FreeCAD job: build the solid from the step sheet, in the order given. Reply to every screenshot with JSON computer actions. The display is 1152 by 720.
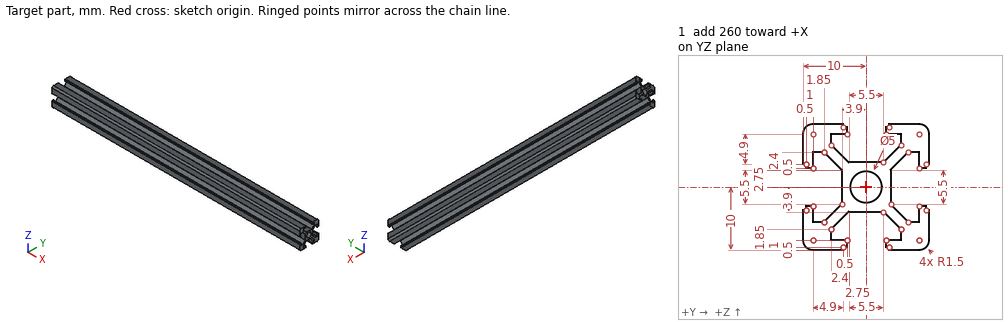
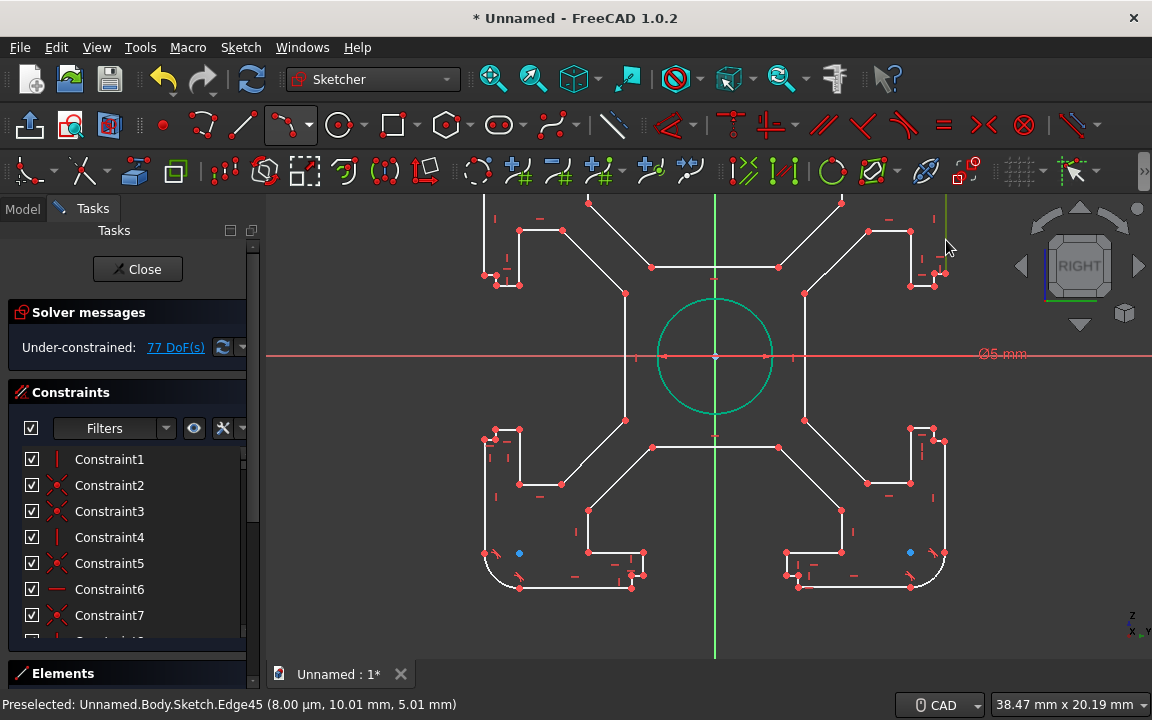
{"action": "scroll", "coordinate": [489, 569], "scroll_direction": "down", "scroll_amount": 2}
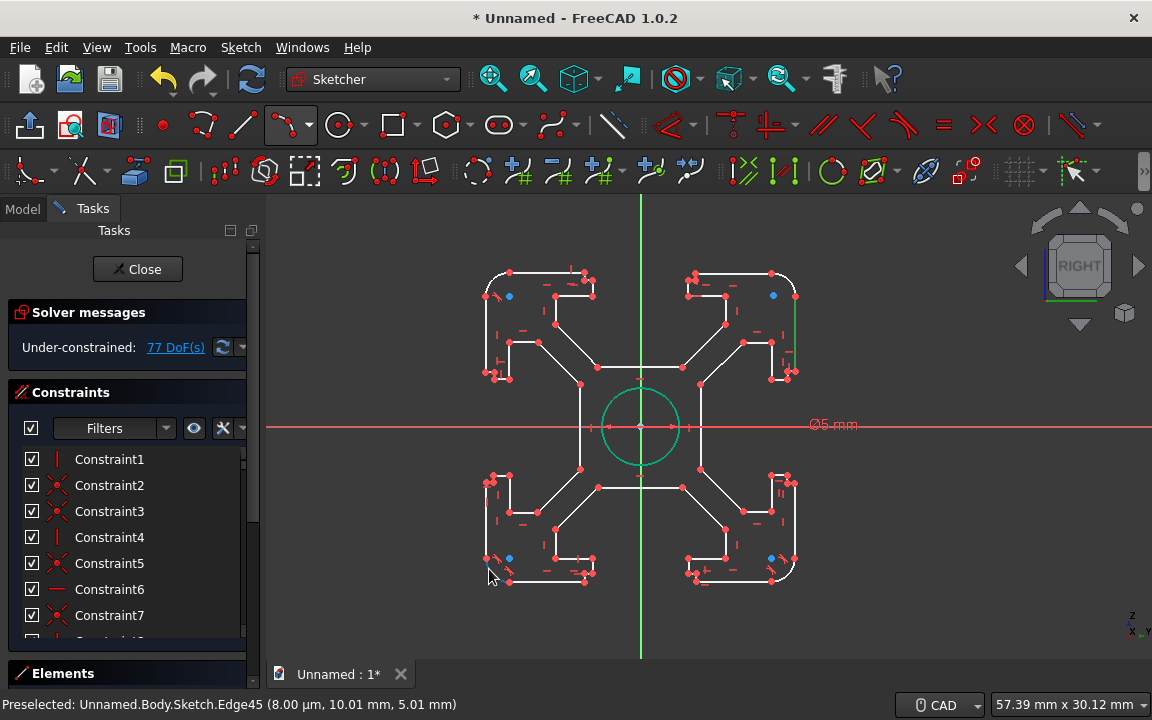
{"action": "scroll", "coordinate": [793, 286], "scroll_direction": "up", "scroll_amount": 2}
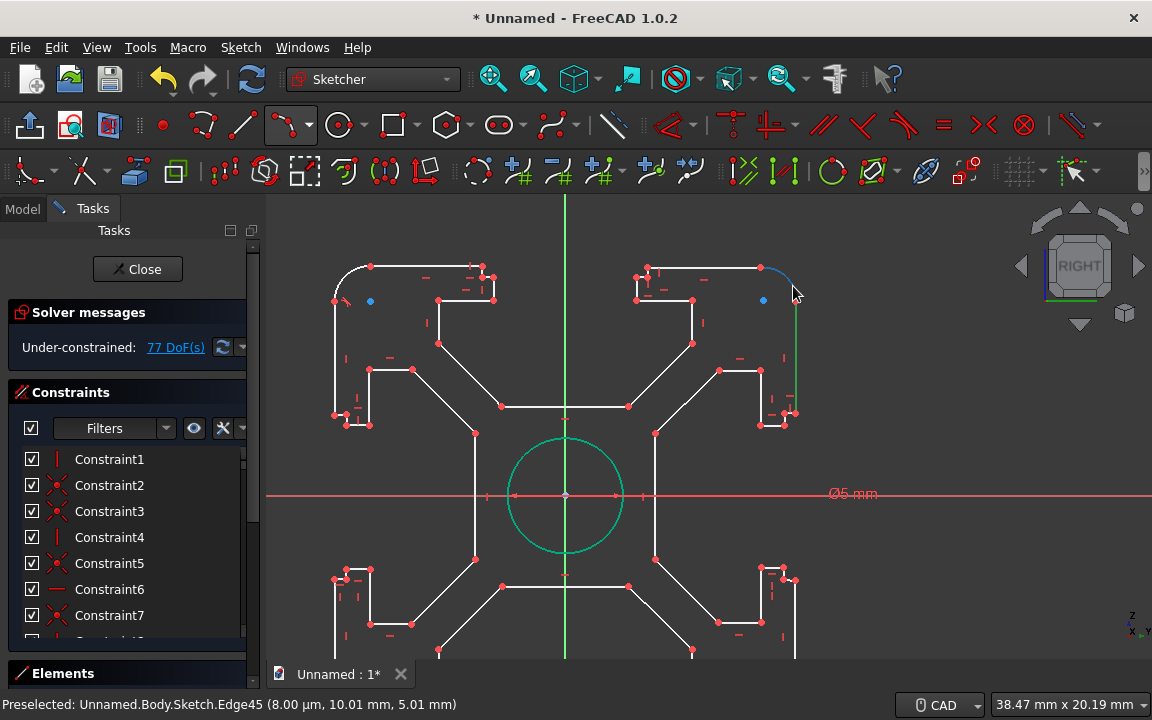
{"action": "left_click", "coordinate": [793, 286]}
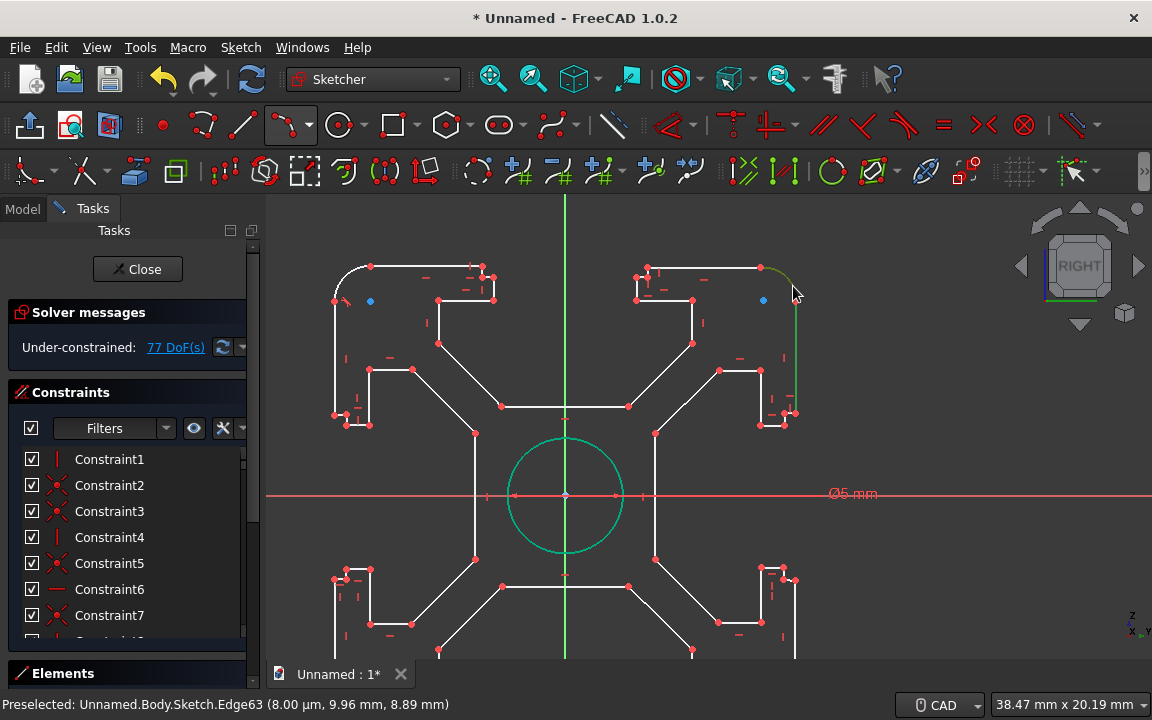
{"action": "key", "text": "t"}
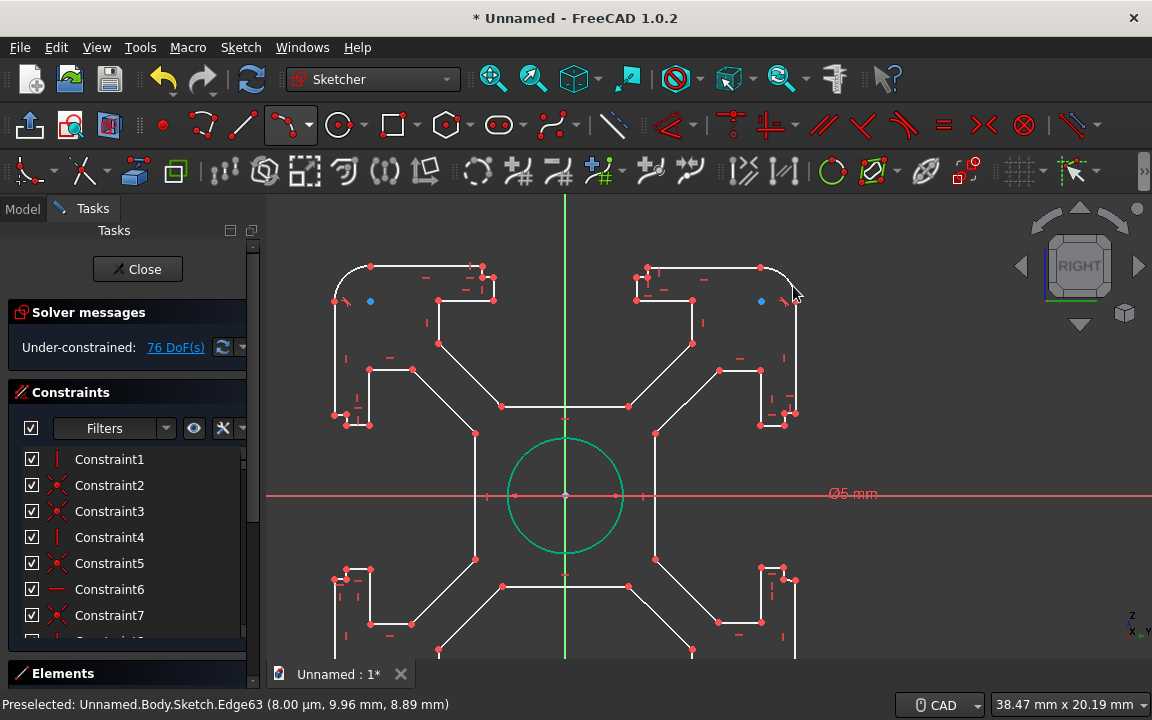
{"action": "left_click", "coordinate": [727, 268]}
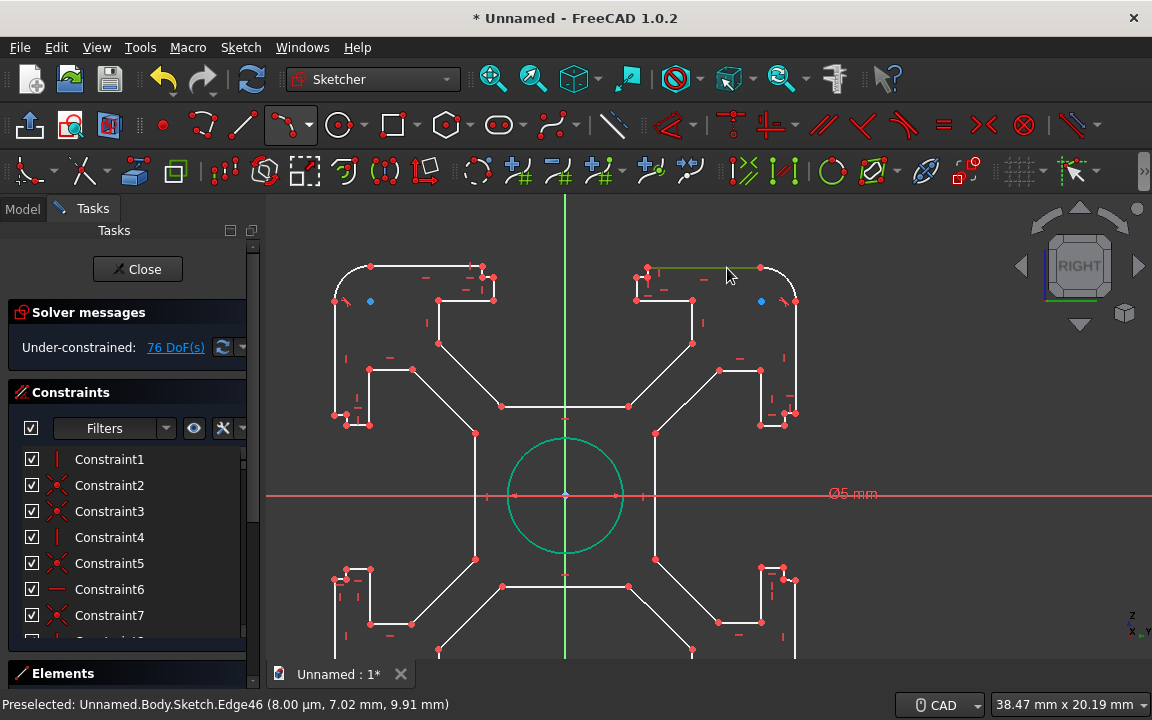
{"action": "left_click", "coordinate": [792, 286]}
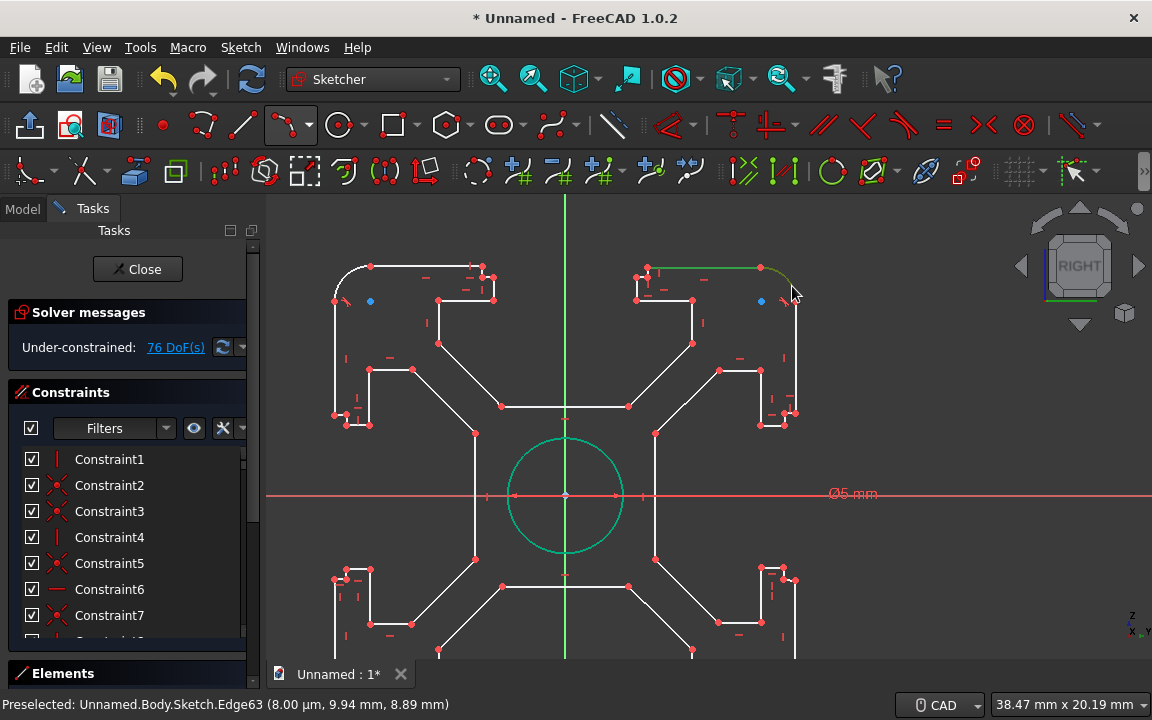
{"action": "key", "text": "t"}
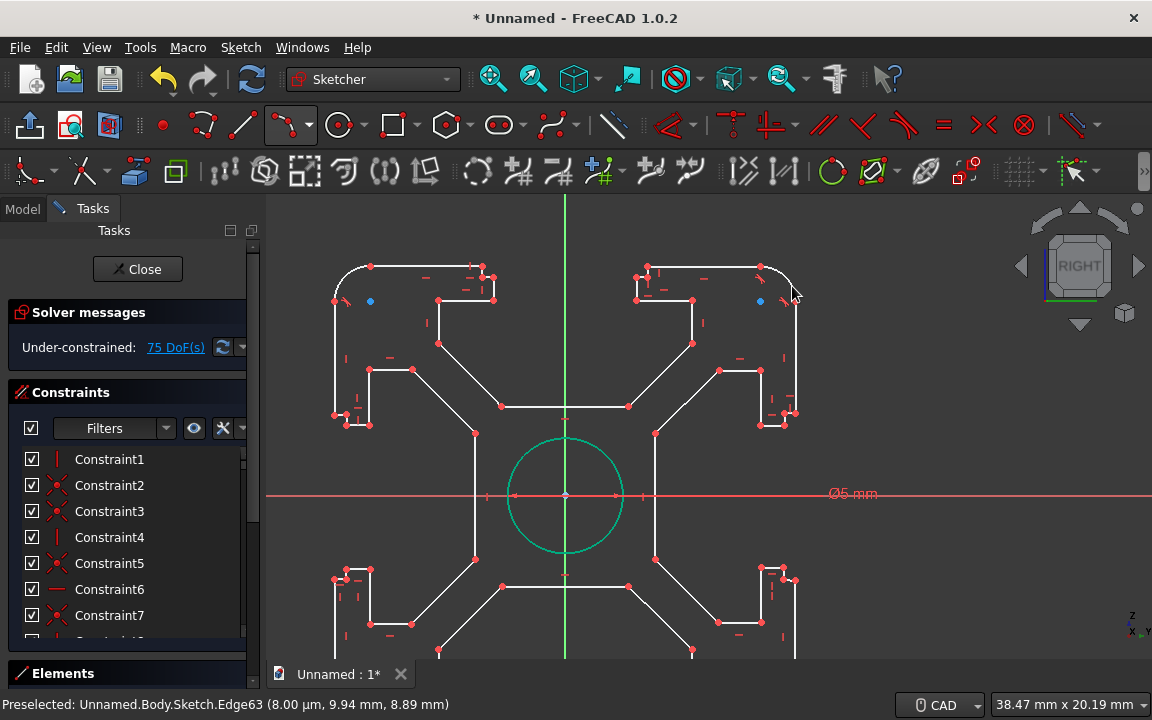
{"action": "left_click", "coordinate": [449, 266]}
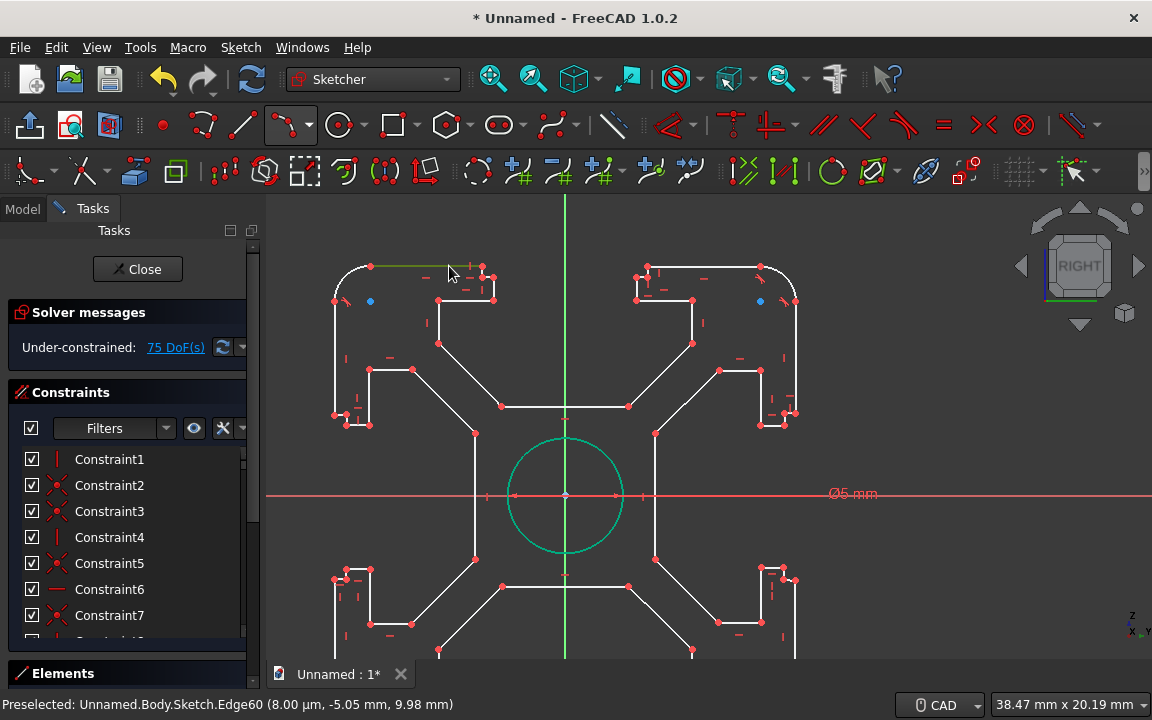
{"action": "left_click", "coordinate": [354, 270]}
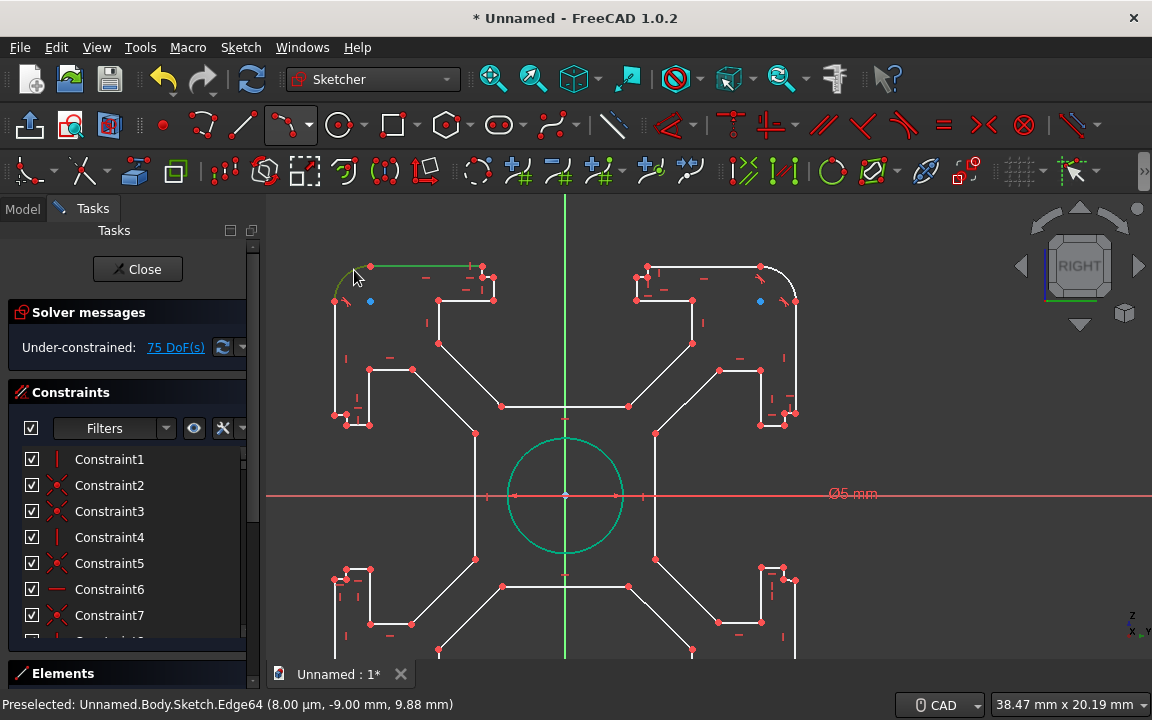
{"action": "key", "text": "t"}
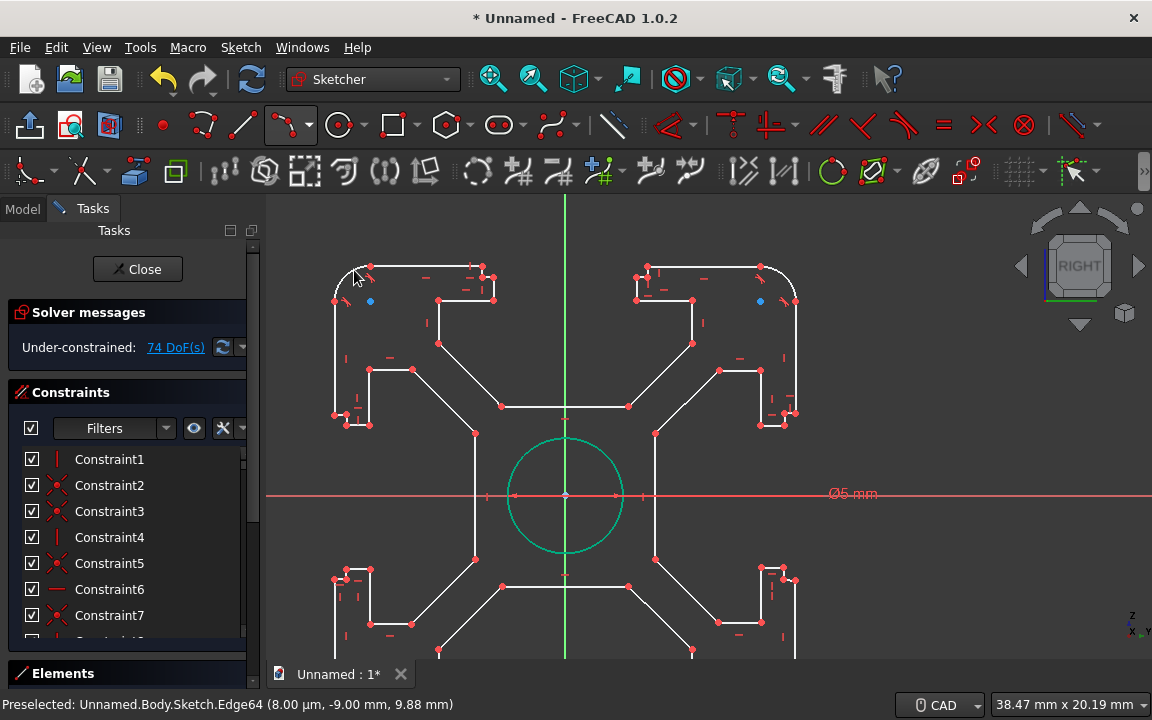
{"action": "scroll", "coordinate": [341, 415], "scroll_direction": "up", "scroll_amount": 5}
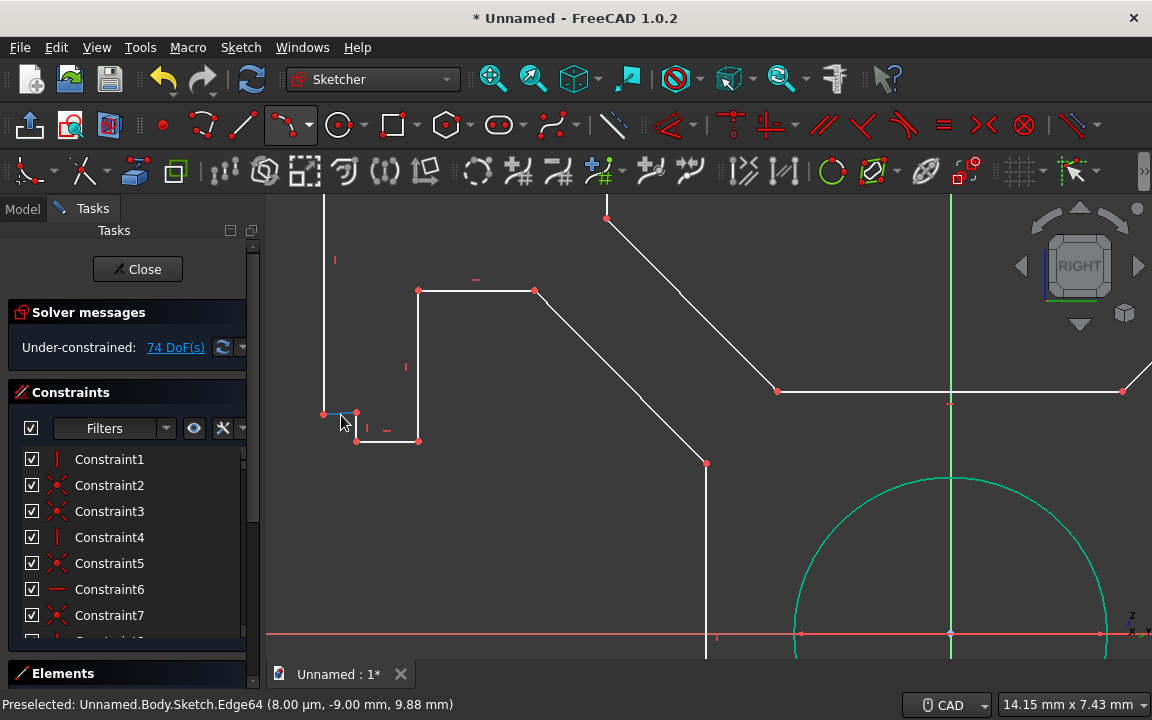
{"action": "left_click", "coordinate": [340, 413]}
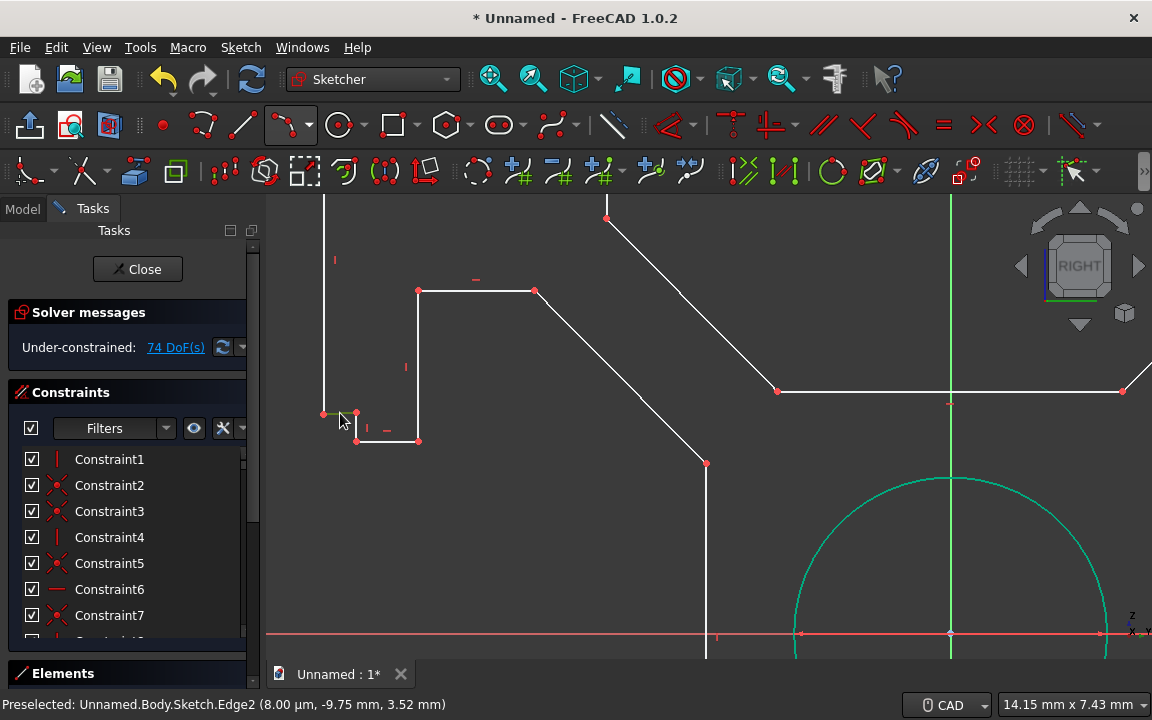
{"action": "key", "text": "h"}